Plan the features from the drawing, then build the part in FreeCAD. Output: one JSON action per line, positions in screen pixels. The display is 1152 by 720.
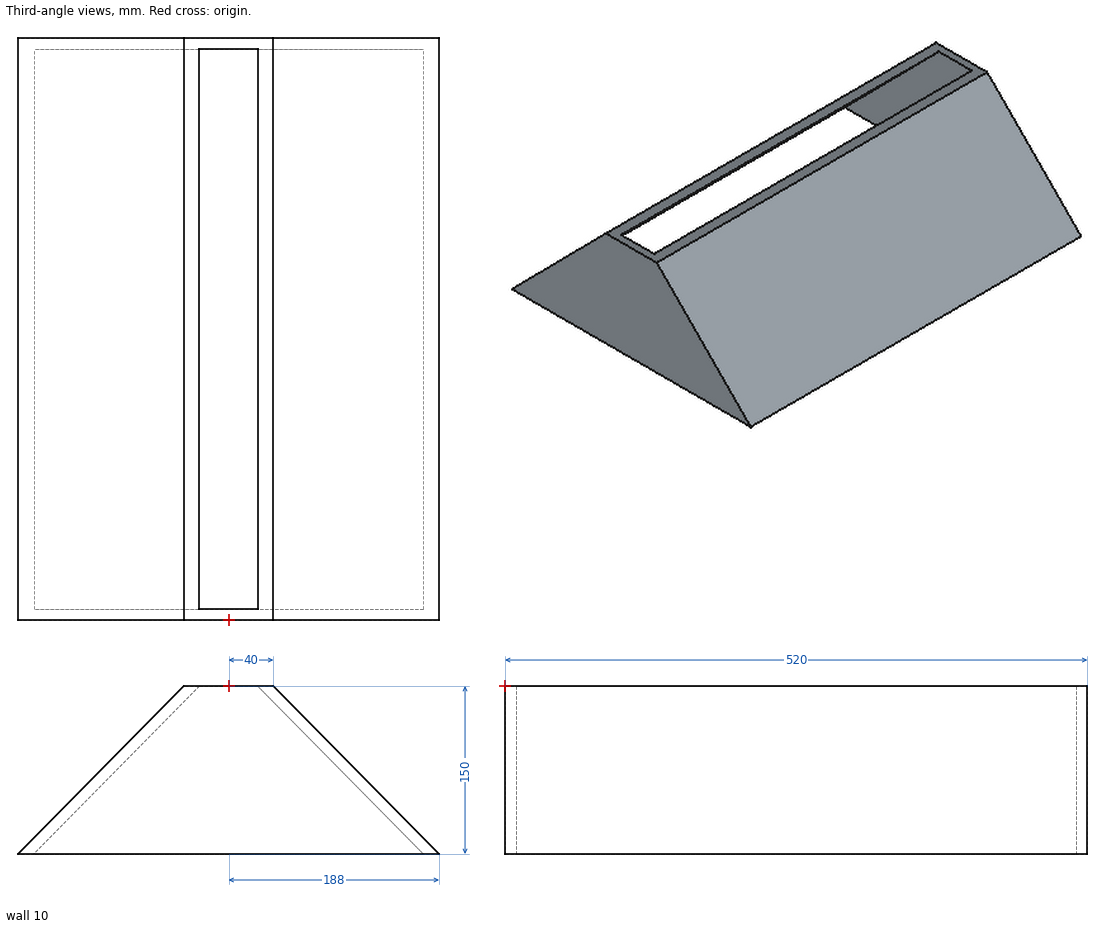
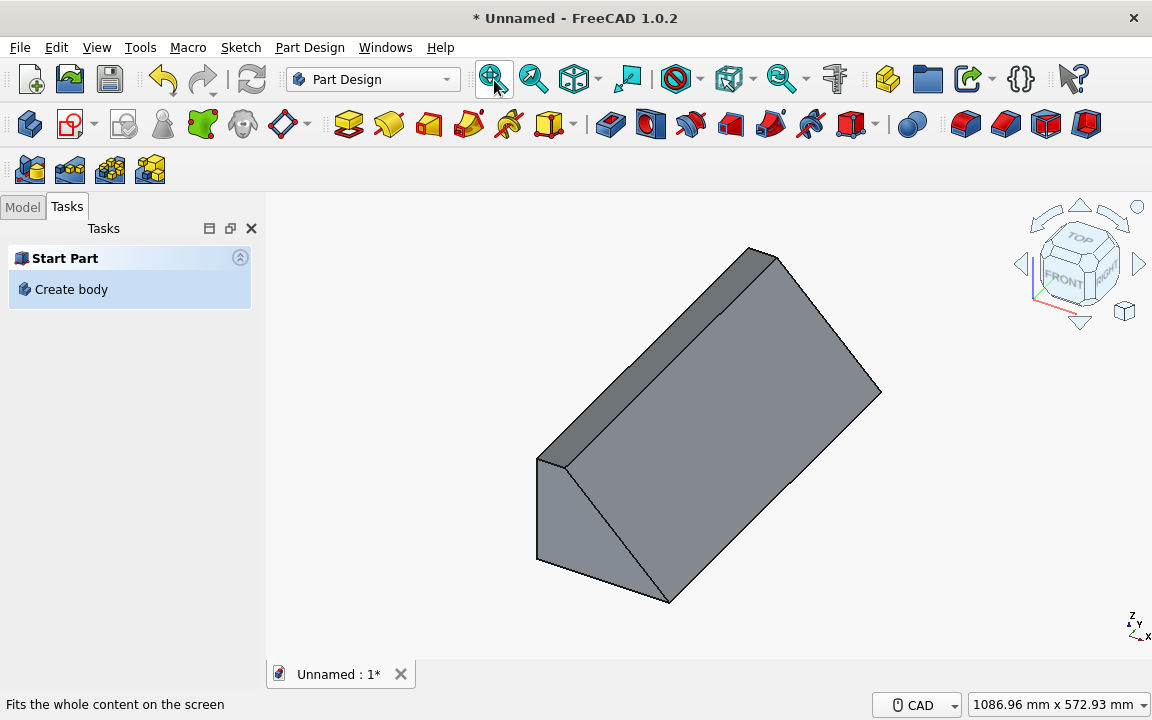
{"action": "left_click", "coordinate": [23, 206]}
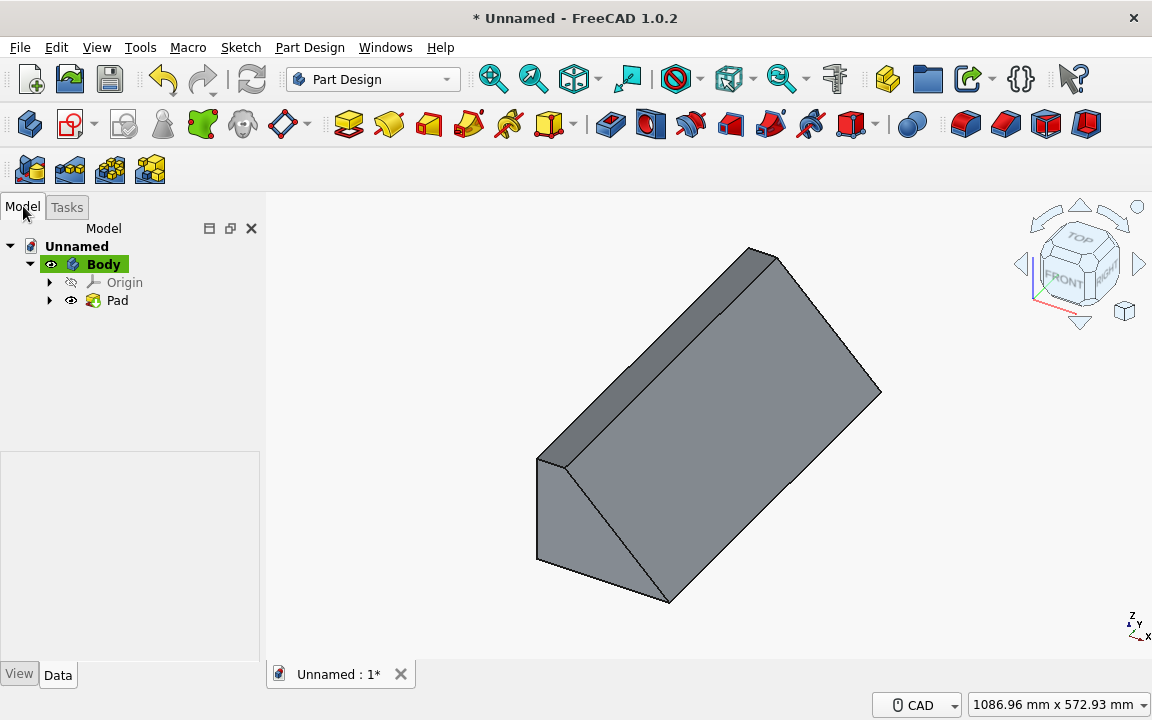
{"action": "left_click", "coordinate": [116, 300]}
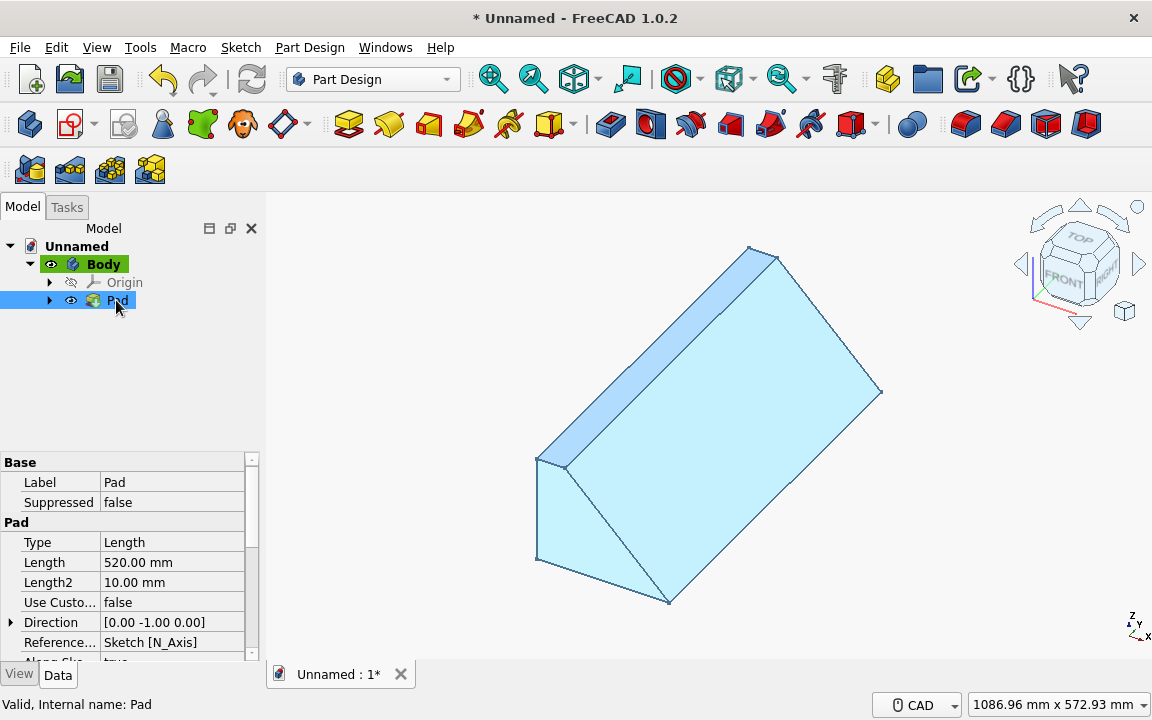
{"action": "left_click", "coordinate": [30, 170]}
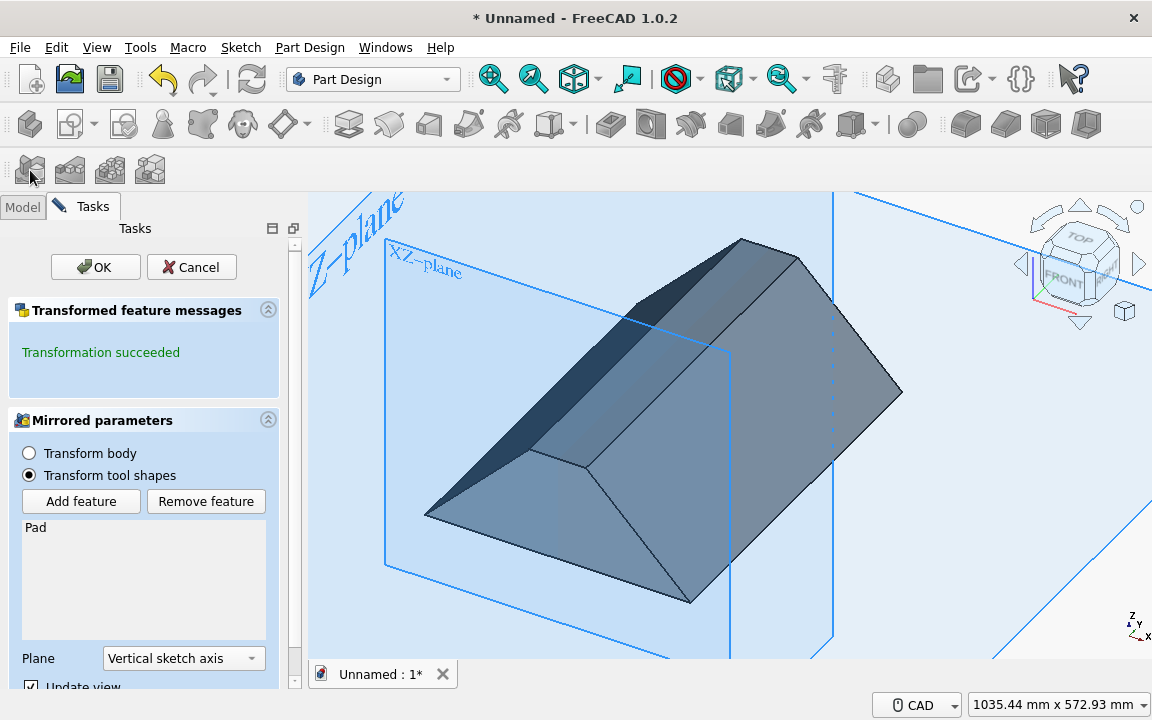
{"action": "left_click", "coordinate": [184, 658]}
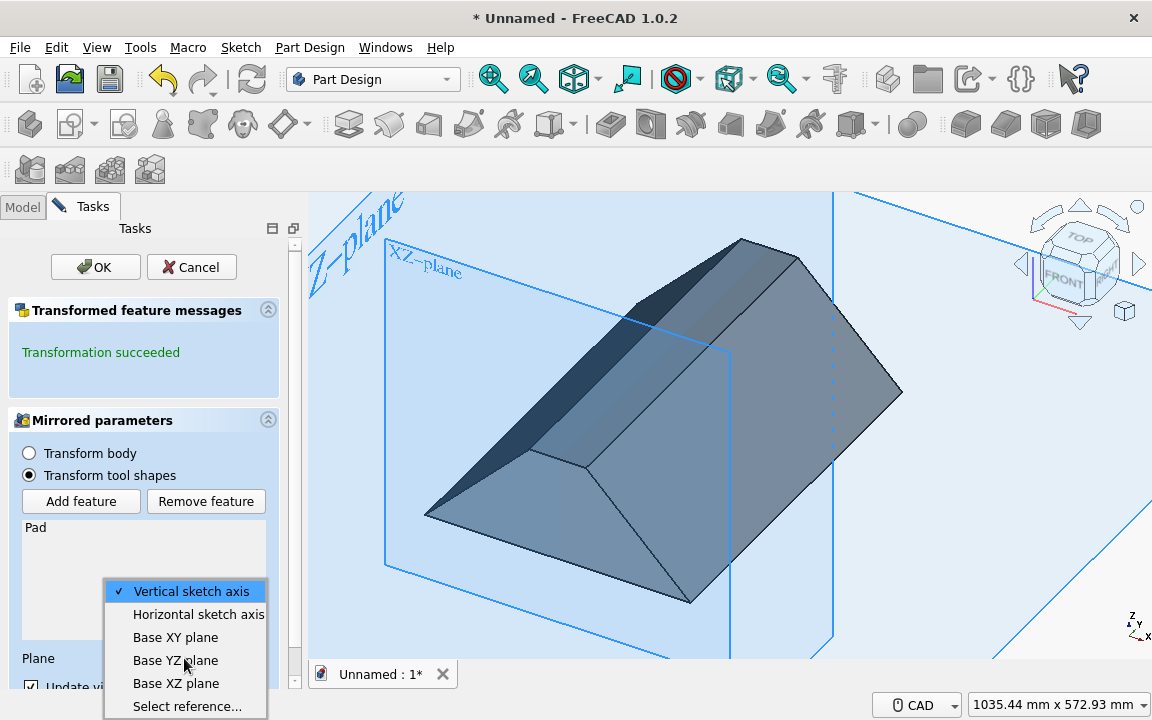
{"action": "left_click", "coordinate": [184, 660]}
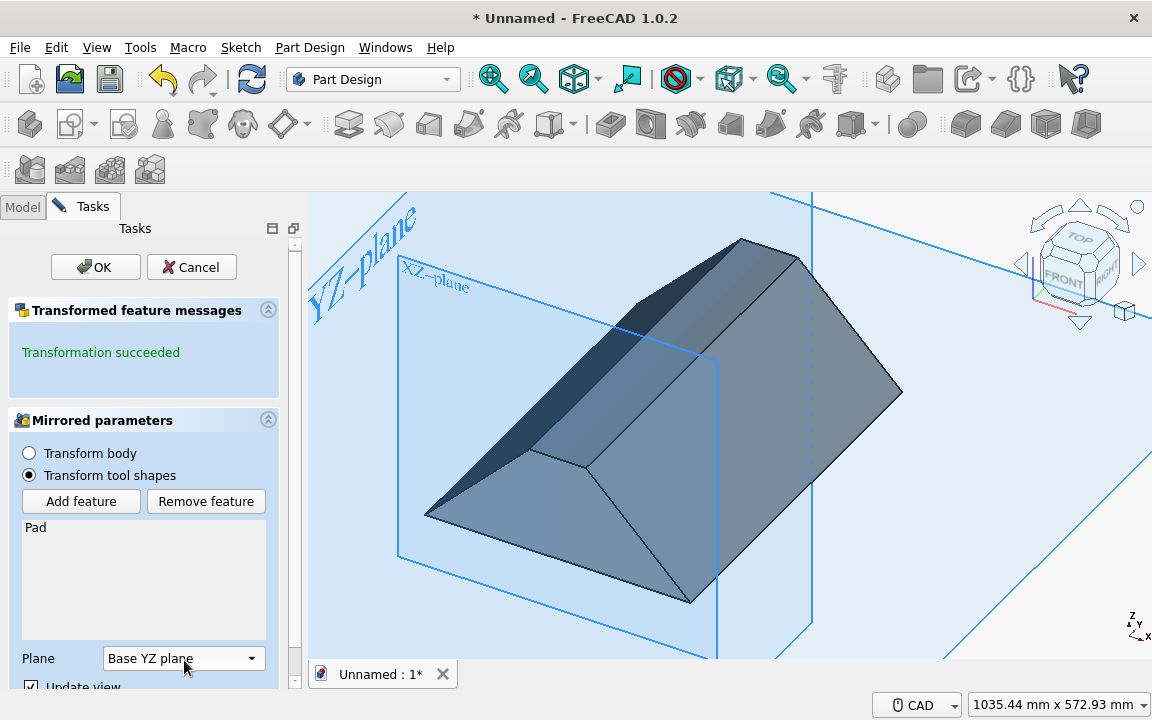
{"action": "left_click", "coordinate": [96, 267]}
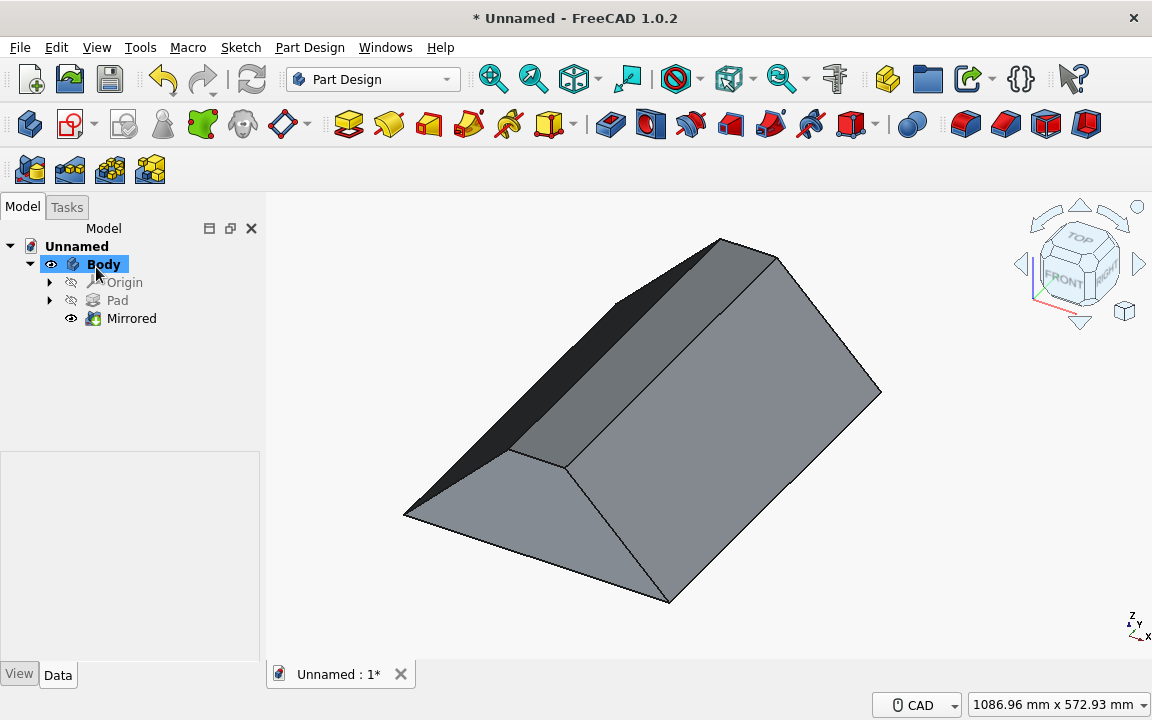
{"action": "left_click", "coordinate": [582, 413]}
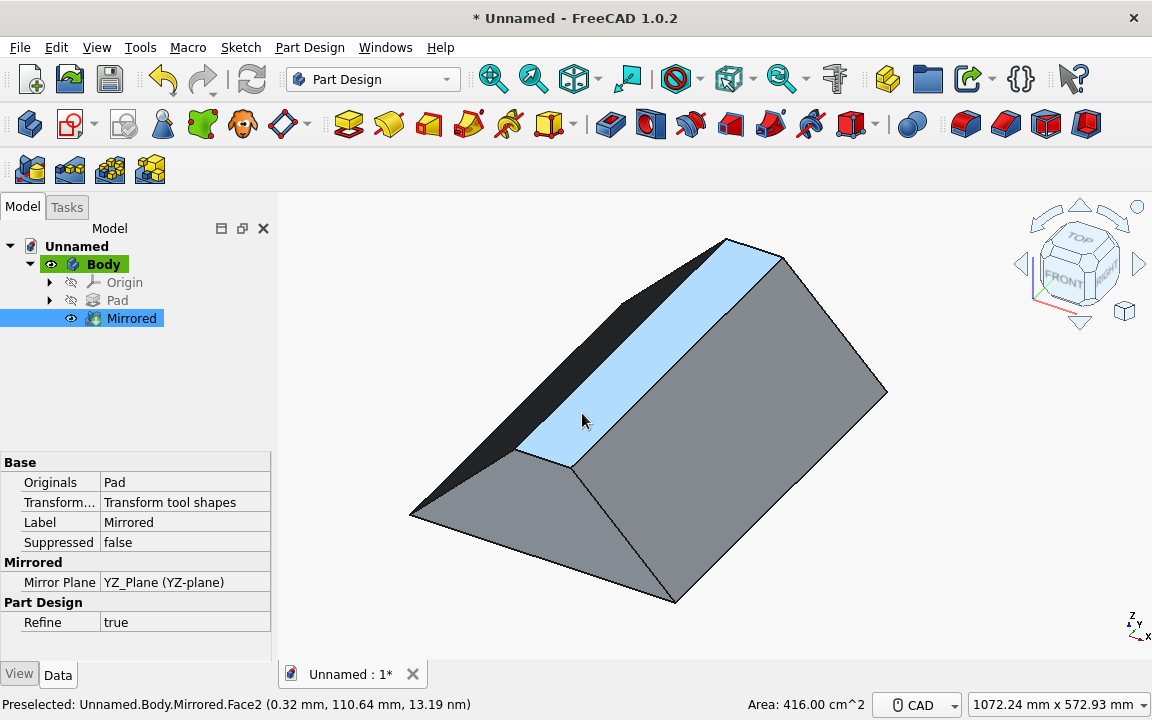
{"action": "key", "text": "0"}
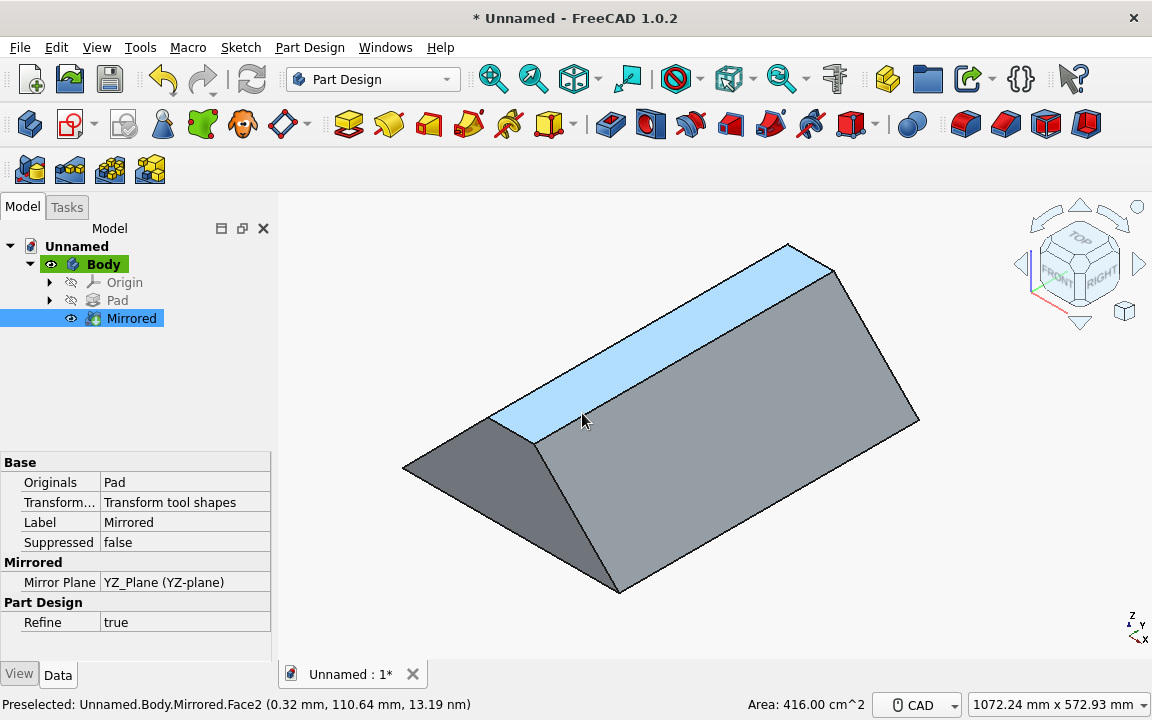
{"action": "key", "text": "2"}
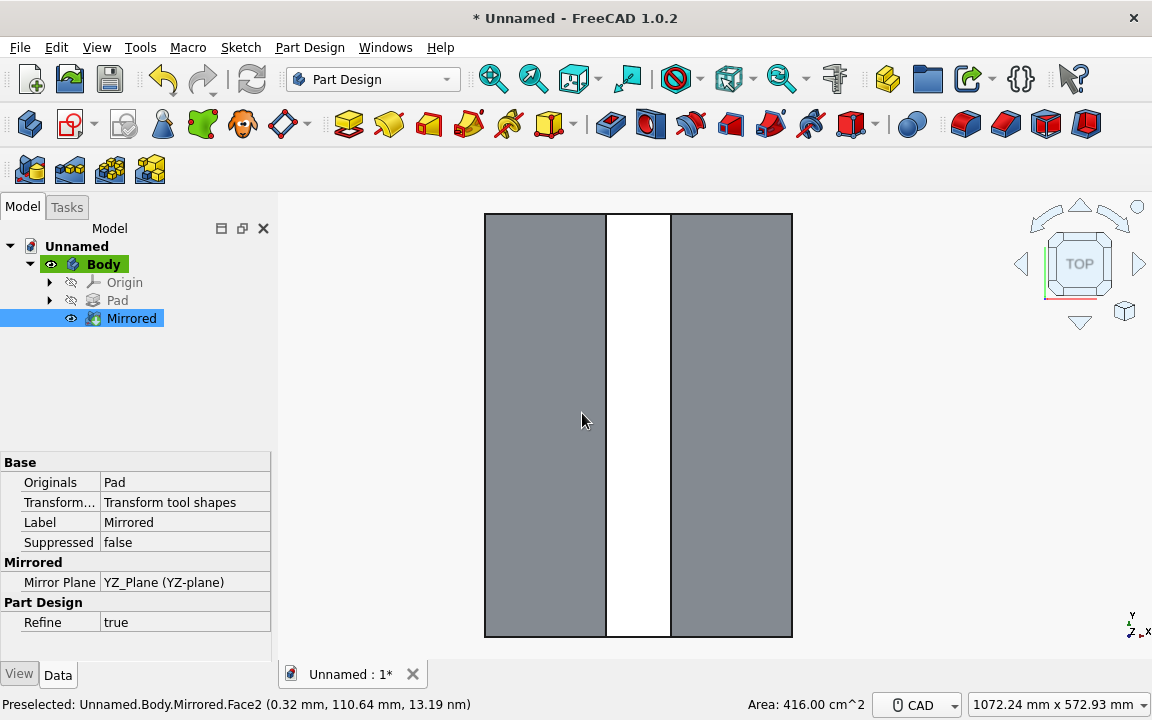
{"action": "key", "text": "1"}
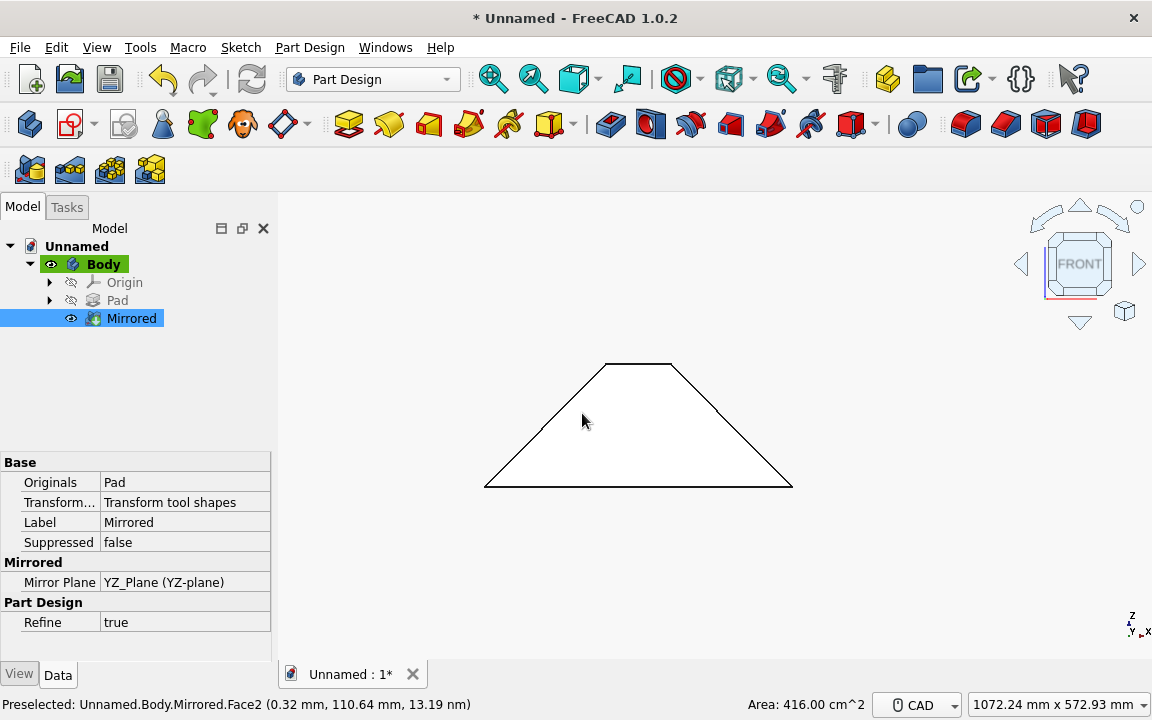
{"action": "key", "text": "v f"}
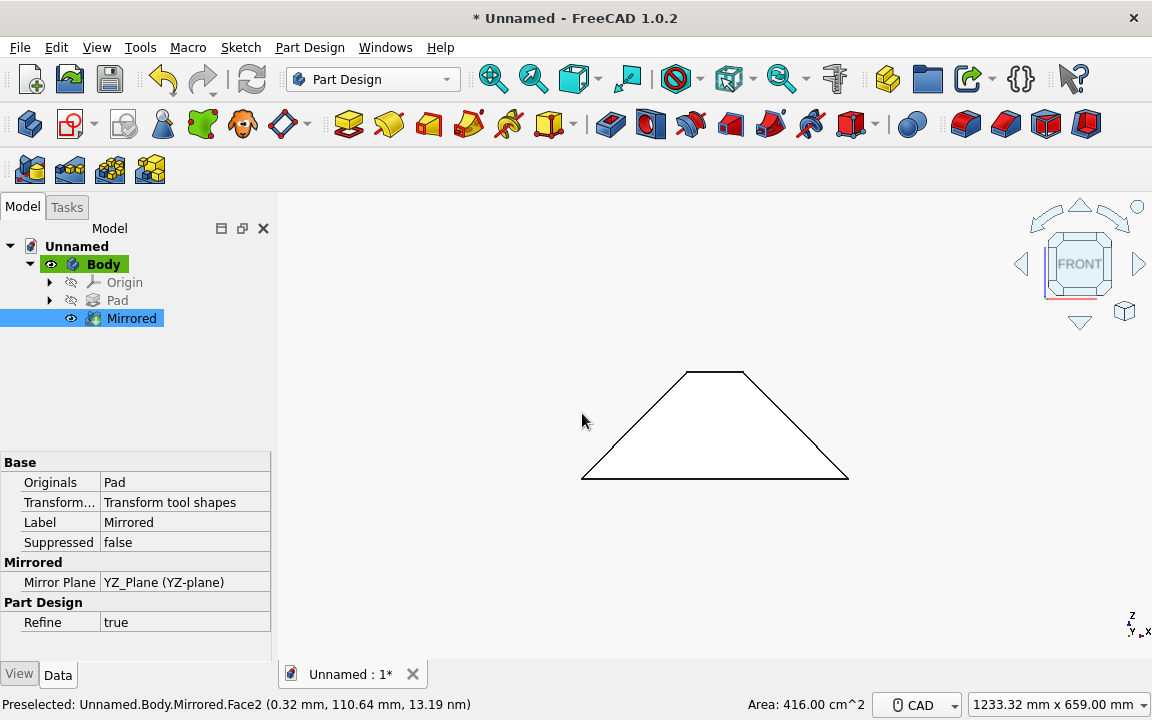
{"action": "key", "text": "3"}